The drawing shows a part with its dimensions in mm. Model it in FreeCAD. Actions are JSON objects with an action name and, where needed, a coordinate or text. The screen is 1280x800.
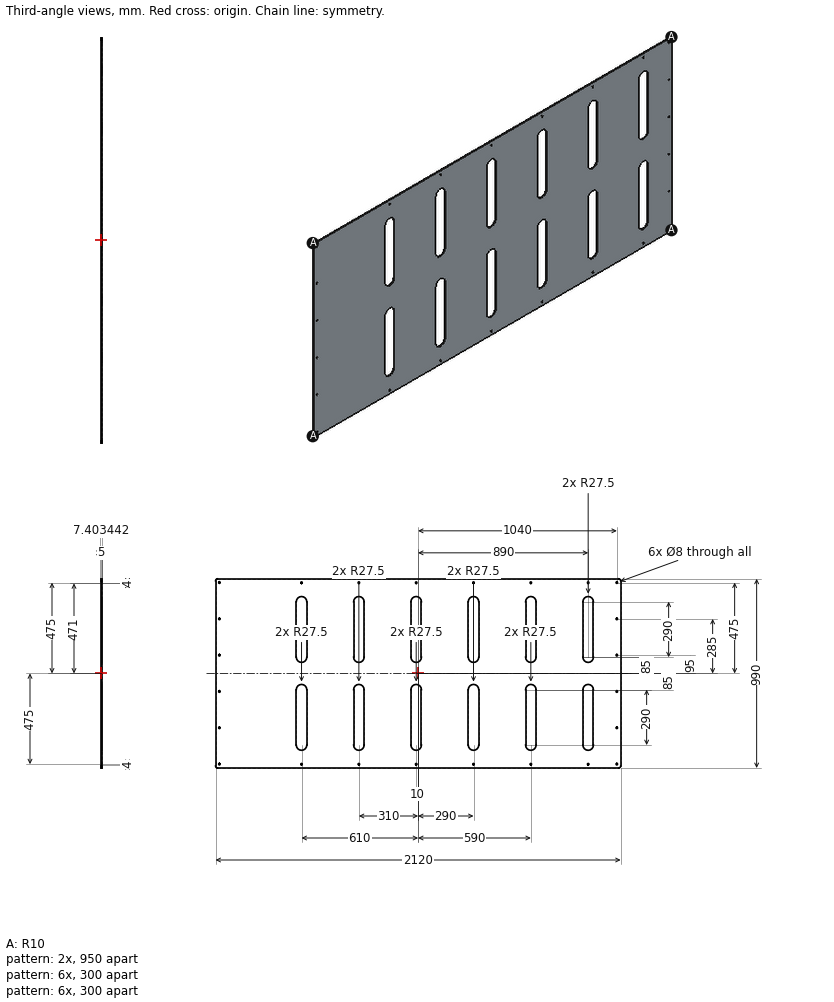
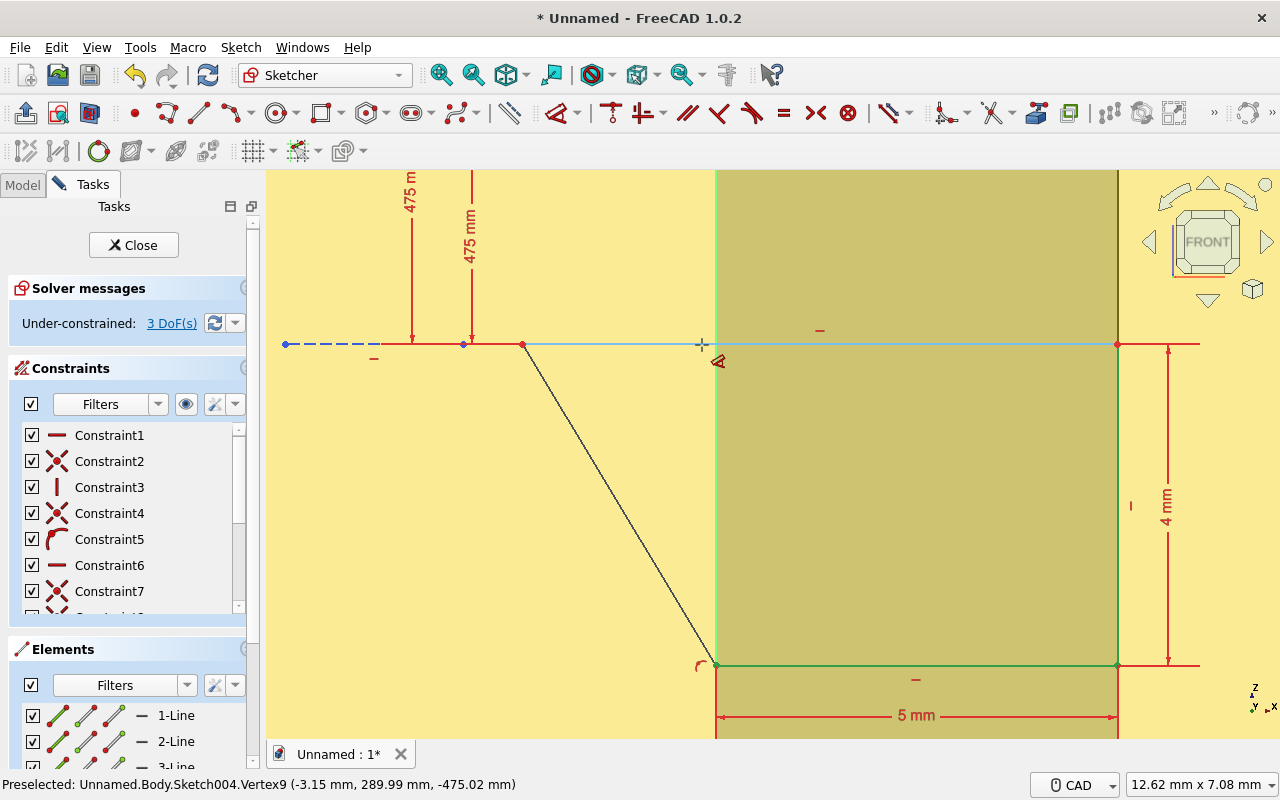
{"action": "left_click", "coordinate": [701, 344]}
{"action": "left_click", "coordinate": [819, 310]}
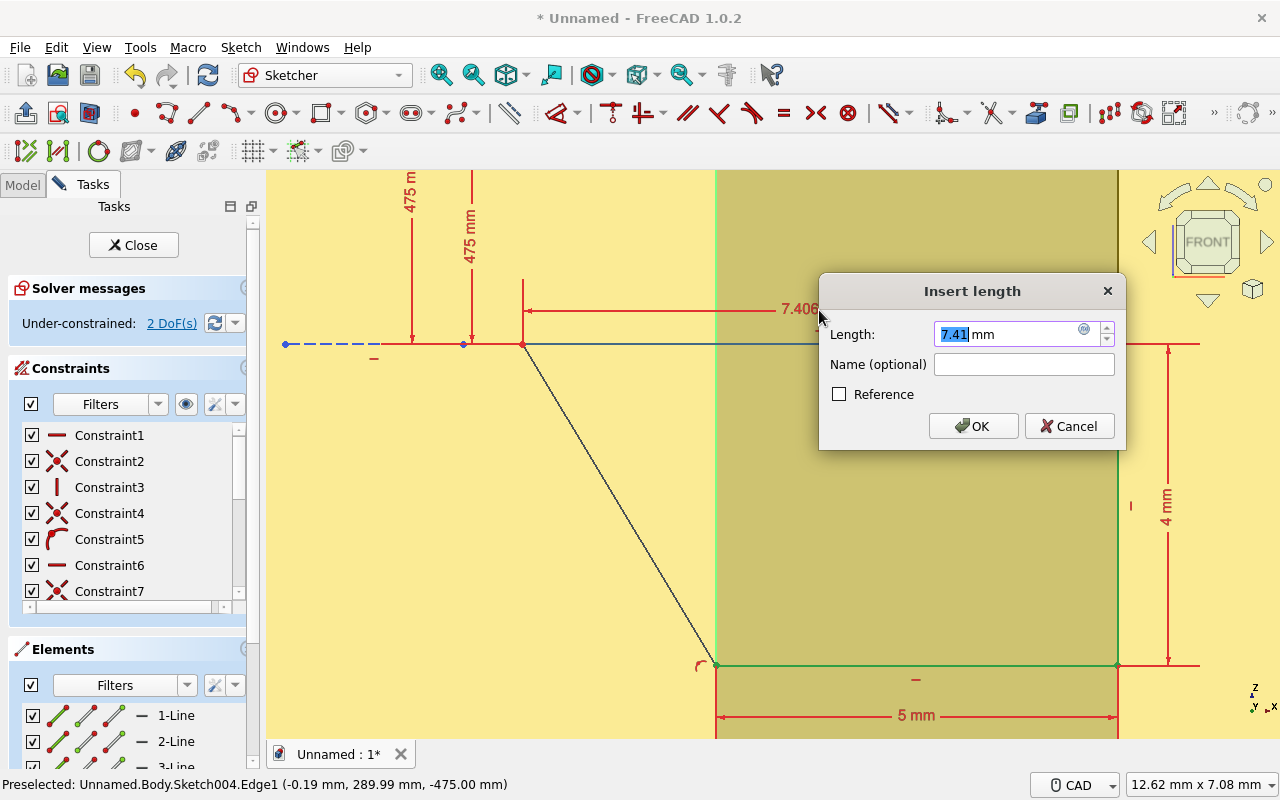
{"action": "type", "text": "7.403442"}
{"action": "key", "text": "Return"}
{"action": "key", "text": "Escape"}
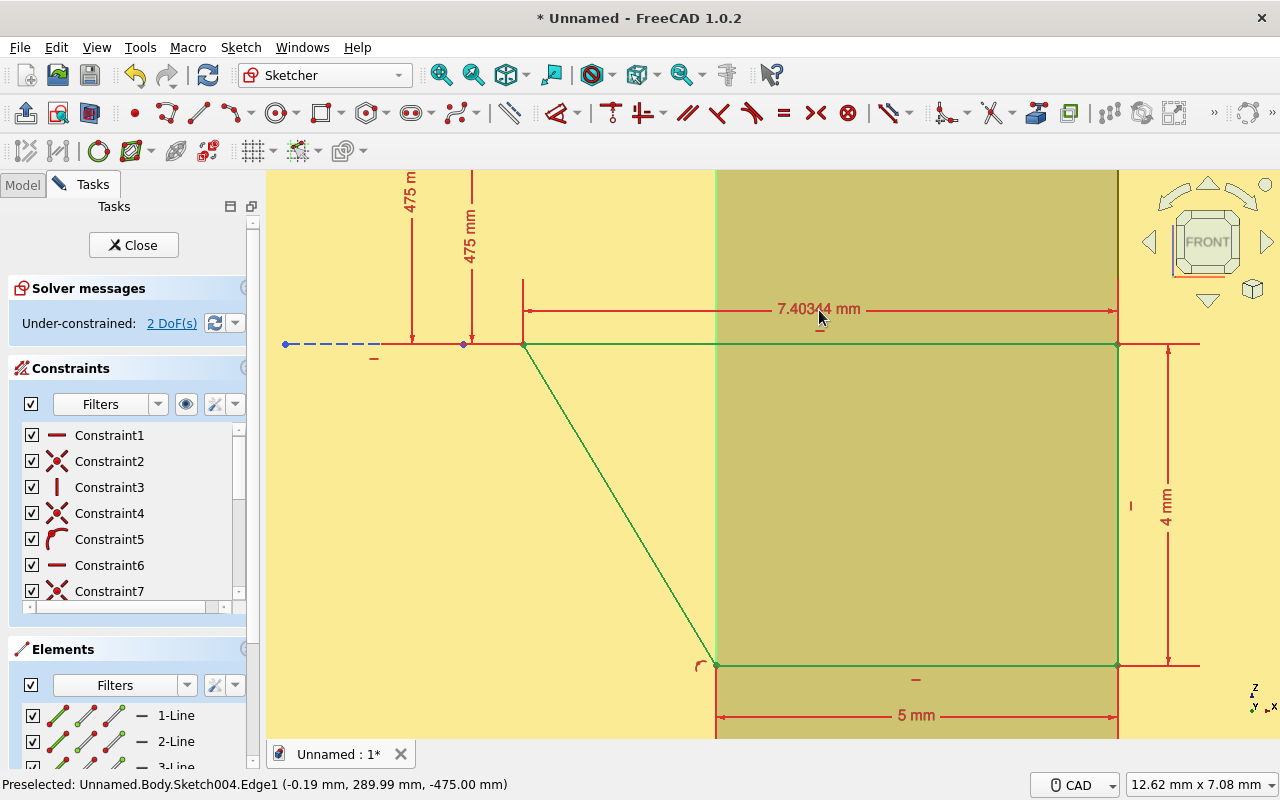
{"action": "left_click", "coordinate": [134, 245]}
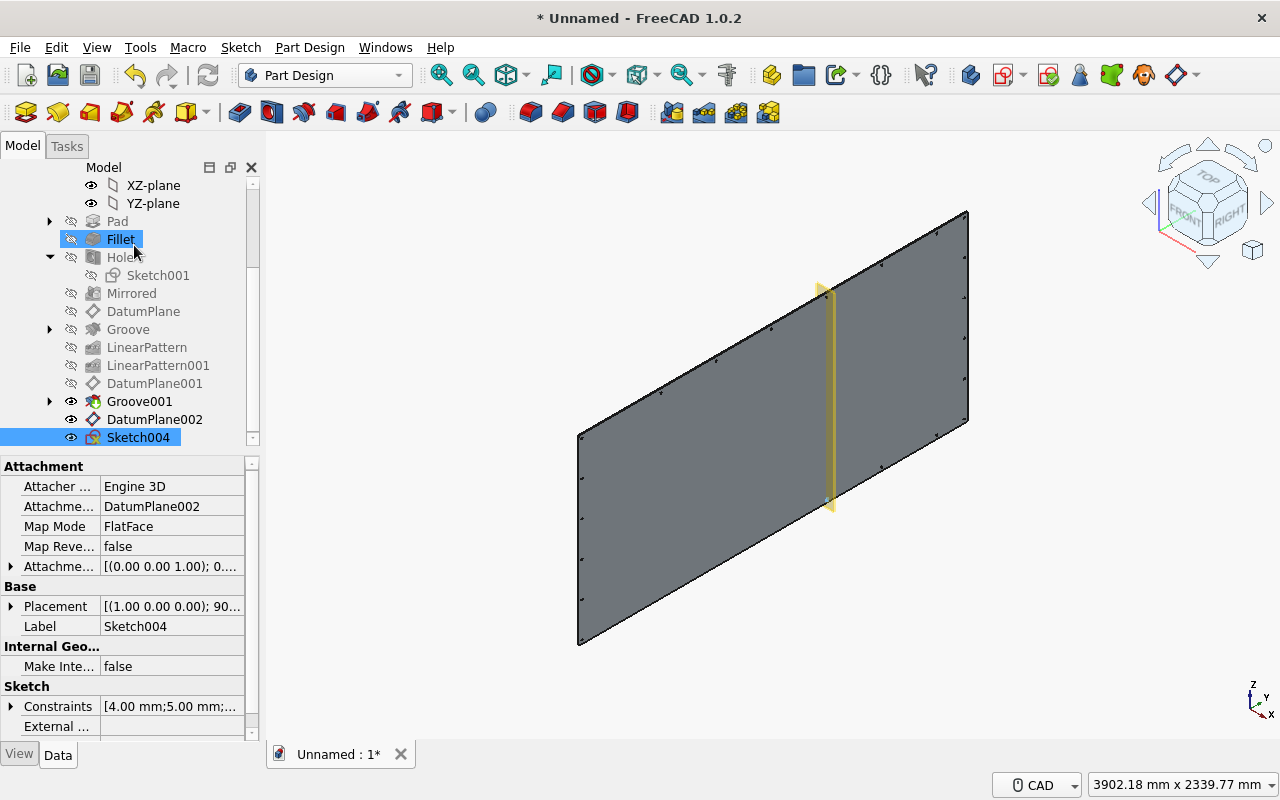
{"action": "left_click", "coordinate": [304, 112]}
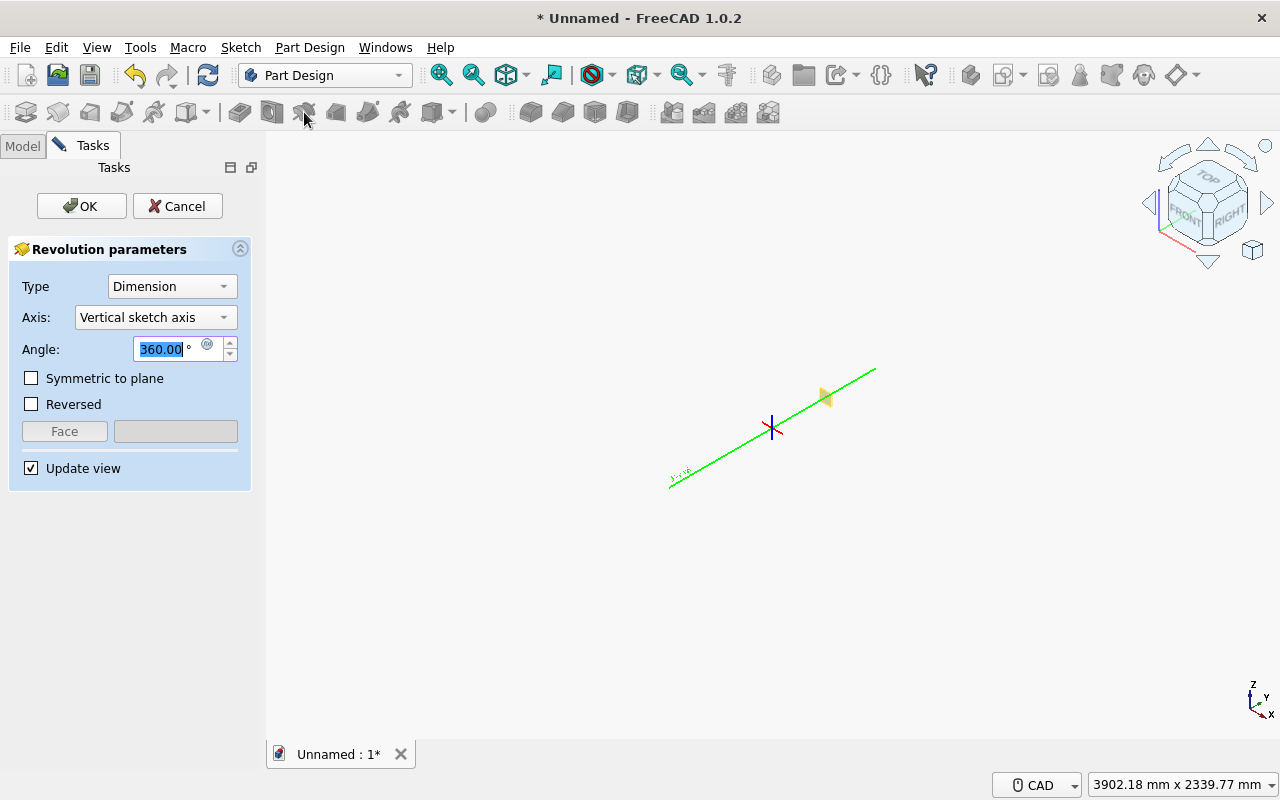
{"action": "left_click", "coordinate": [156, 318]}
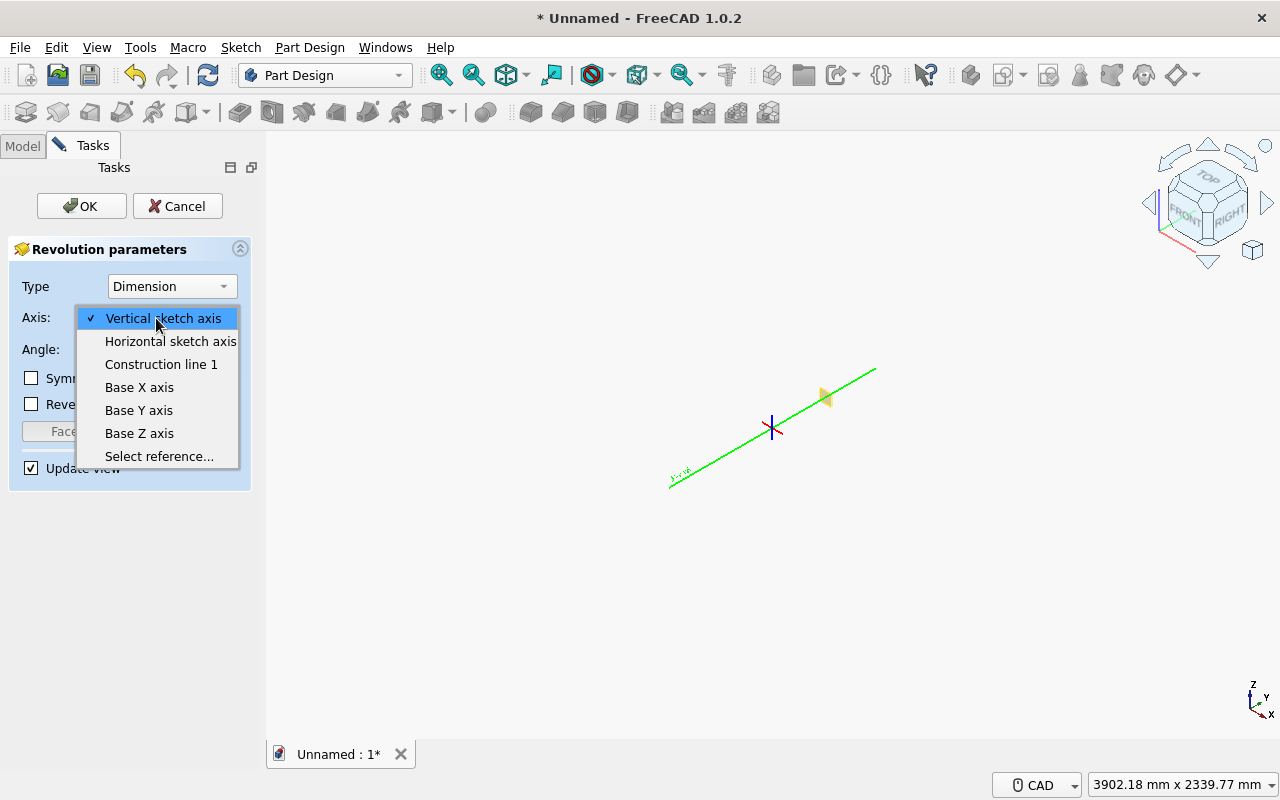
{"action": "left_click", "coordinate": [156, 364]}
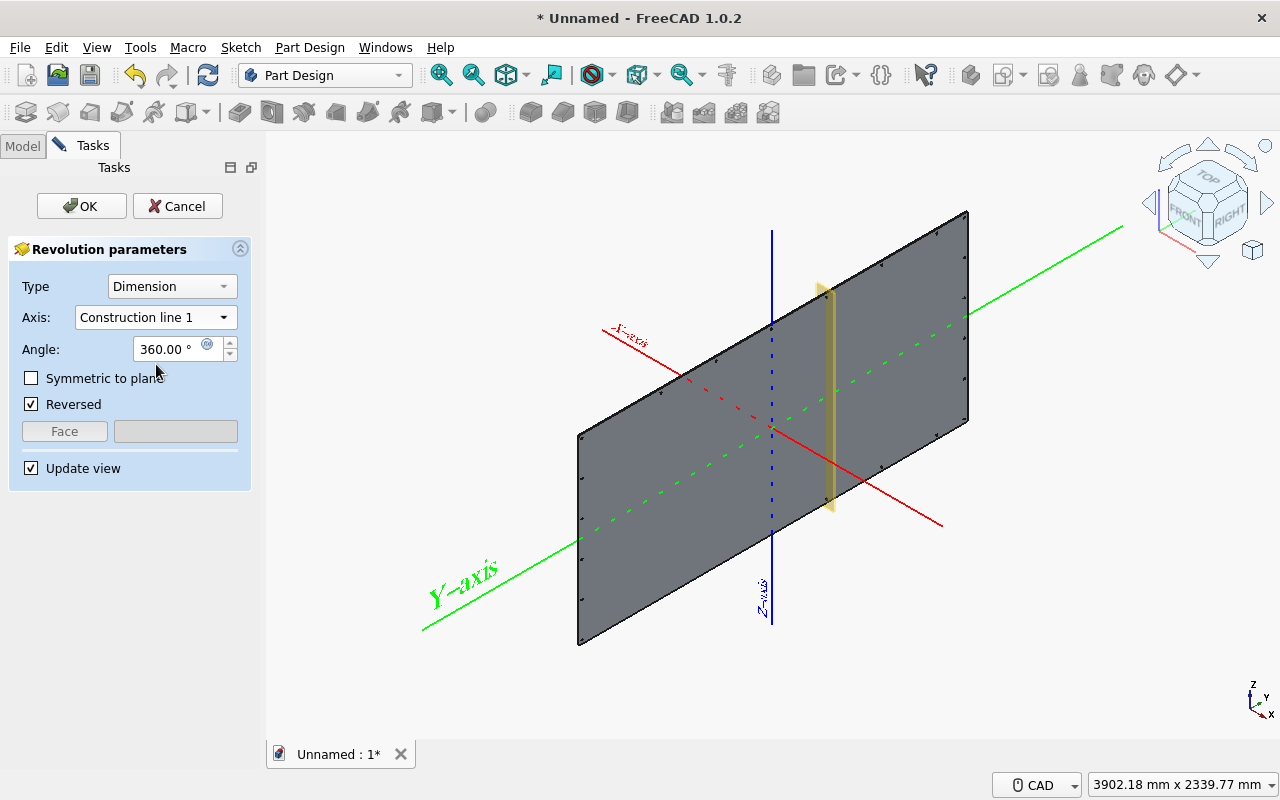
{"action": "left_click", "coordinate": [82, 206]}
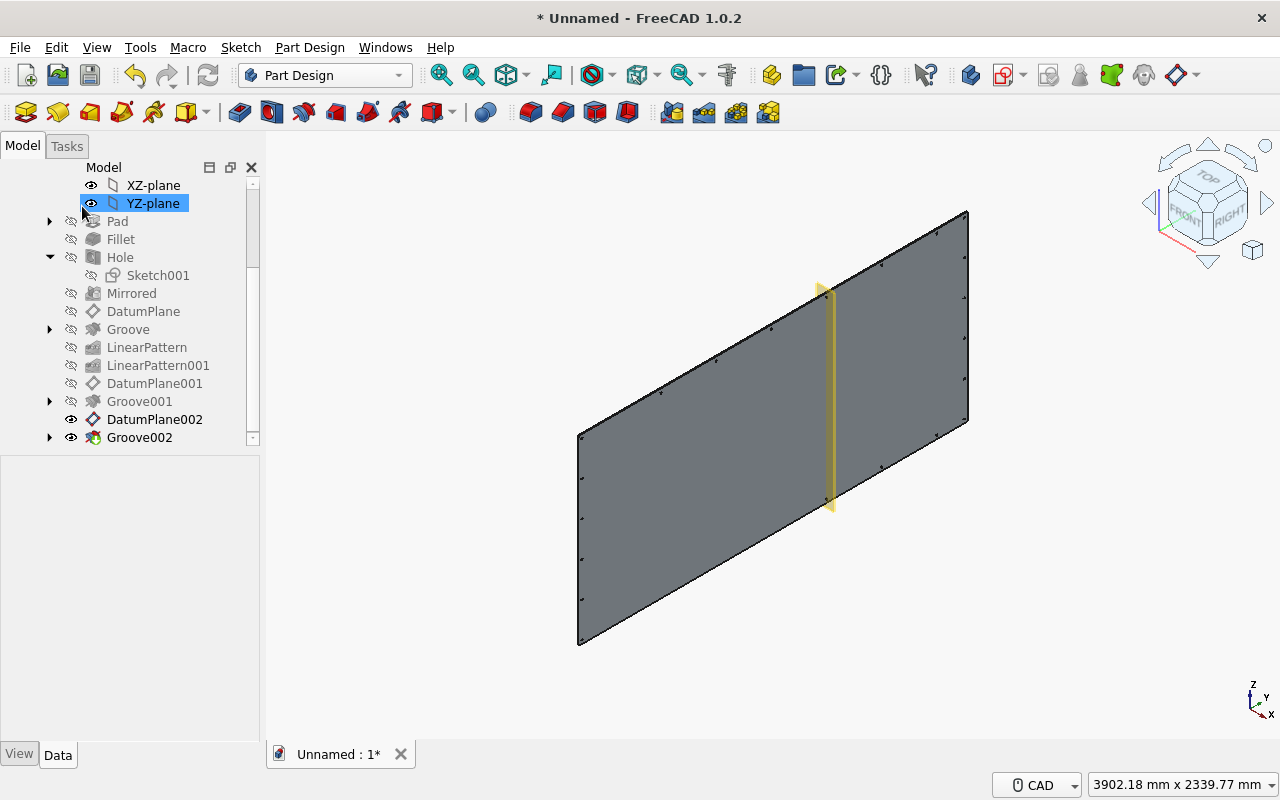
{"action": "left_click", "coordinate": [116, 419]}
{"action": "key", "text": "space"}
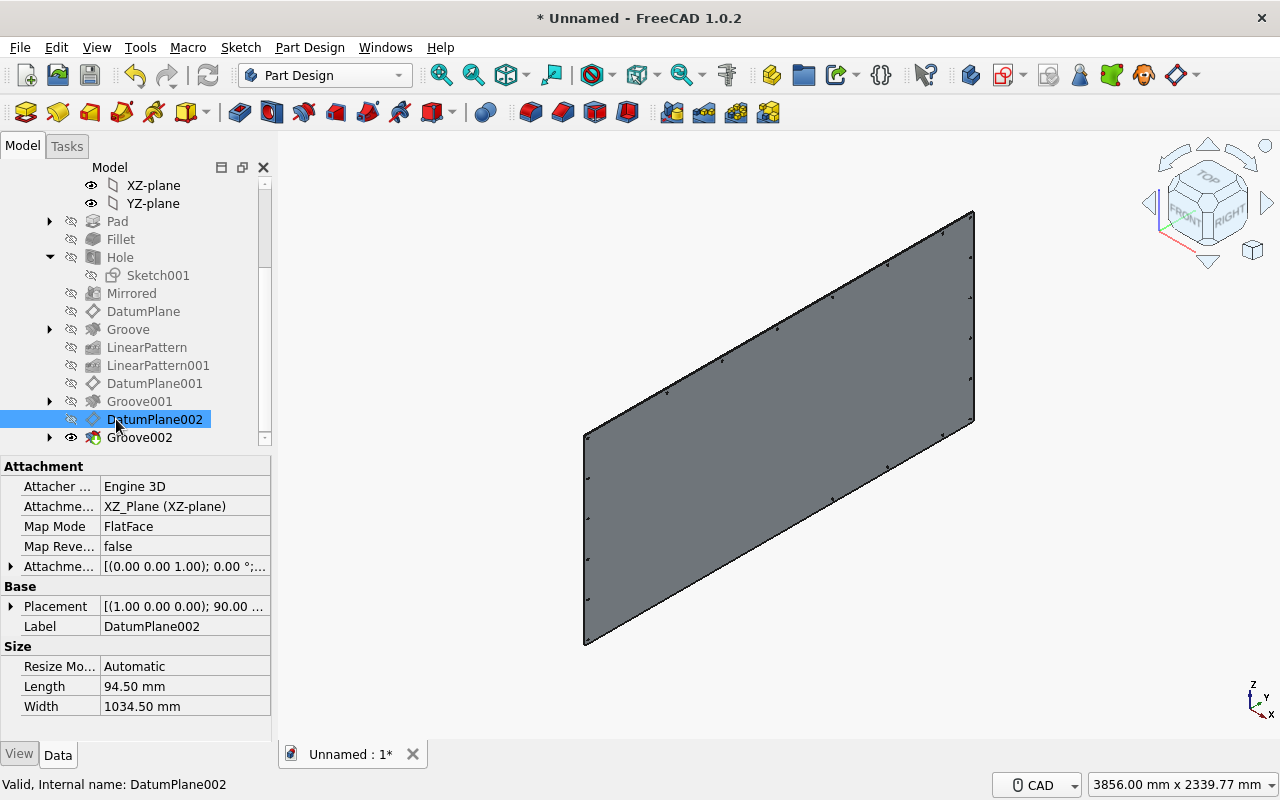
{"action": "scroll", "coordinate": [160, 307], "scroll_direction": "down", "scroll_amount": 3}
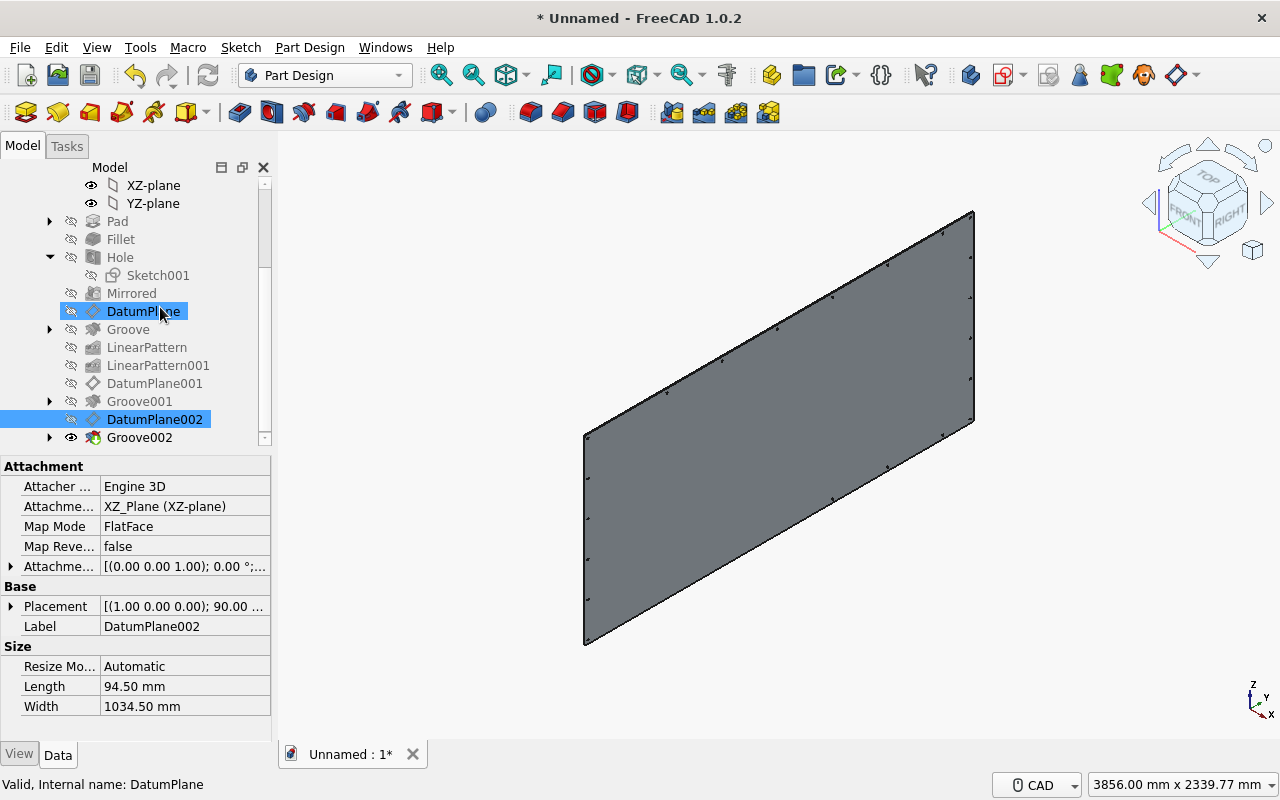
{"action": "scroll", "coordinate": [160, 307], "scroll_direction": "up", "scroll_amount": 15}